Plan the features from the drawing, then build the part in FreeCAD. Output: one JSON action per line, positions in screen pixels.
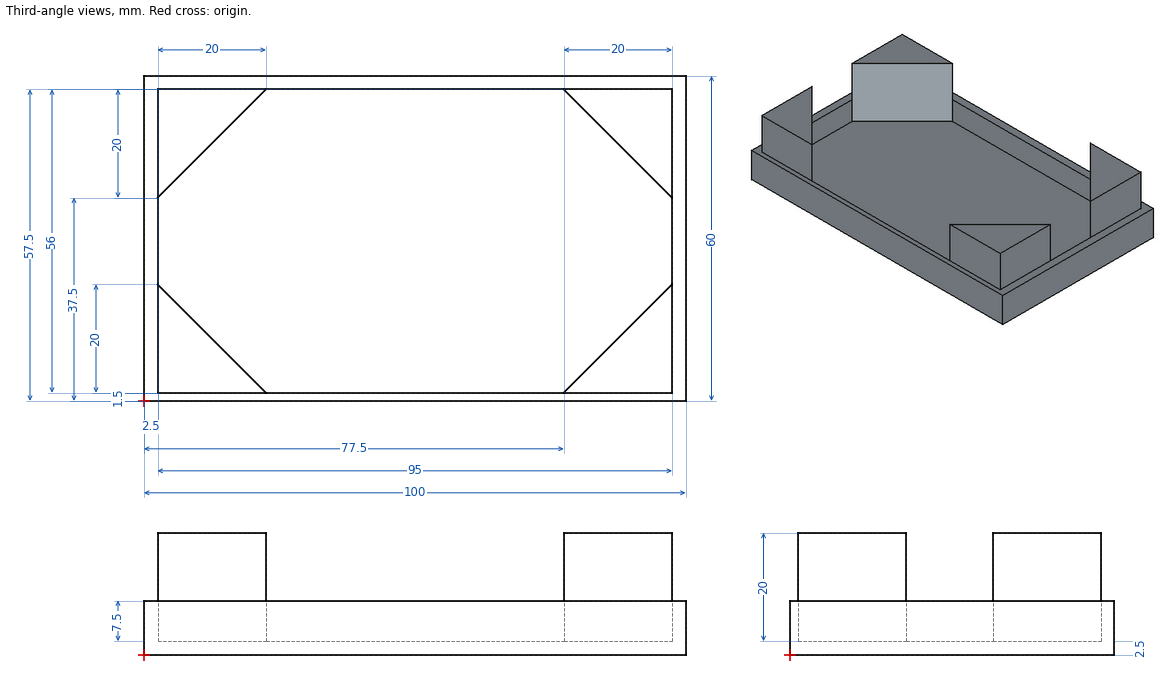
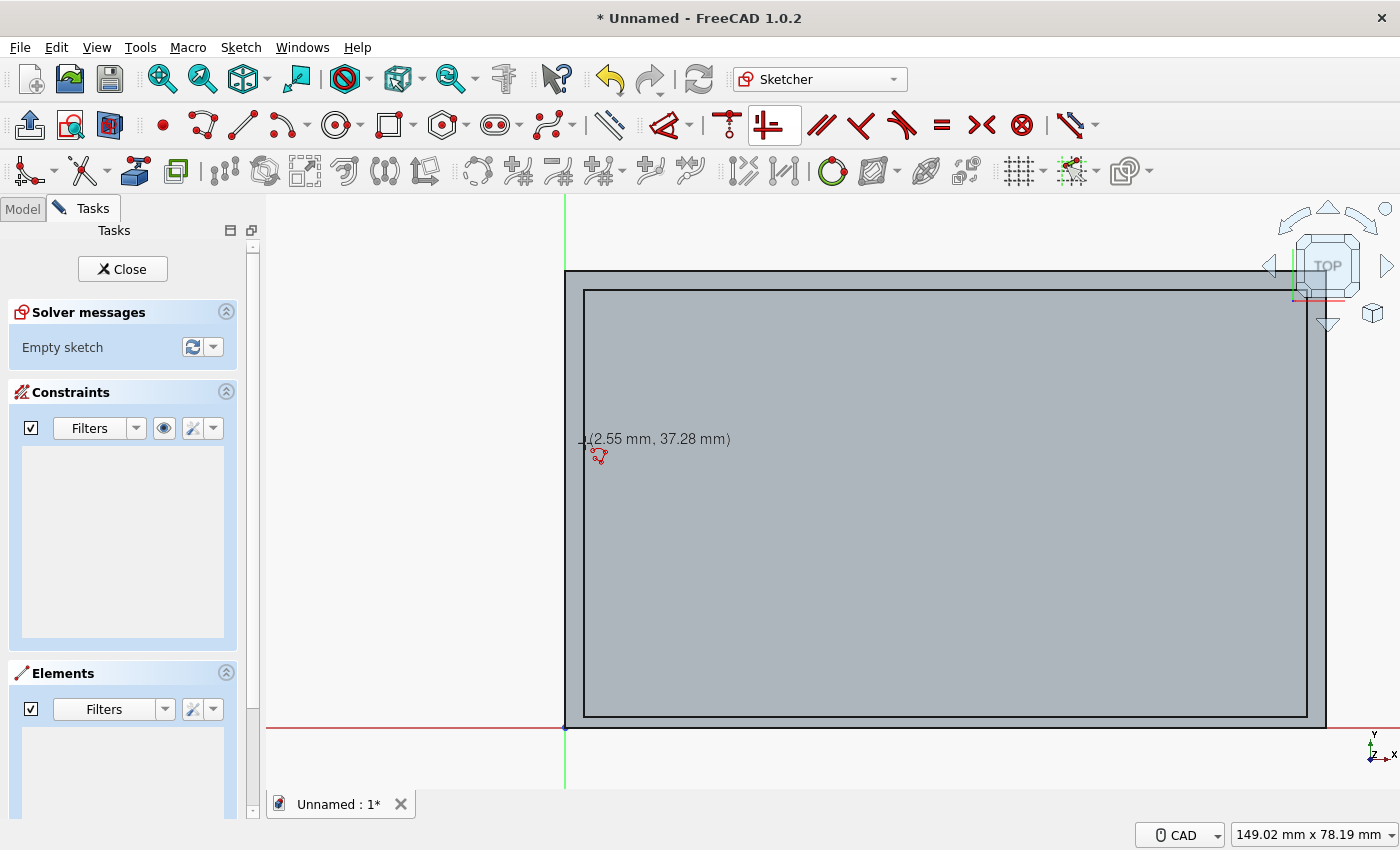
{"action": "left_click", "coordinate": [584, 443]}
{"action": "left_click", "coordinate": [737, 290]}
{"action": "left_click", "coordinate": [584, 290]}
{"action": "left_click", "coordinate": [584, 444]}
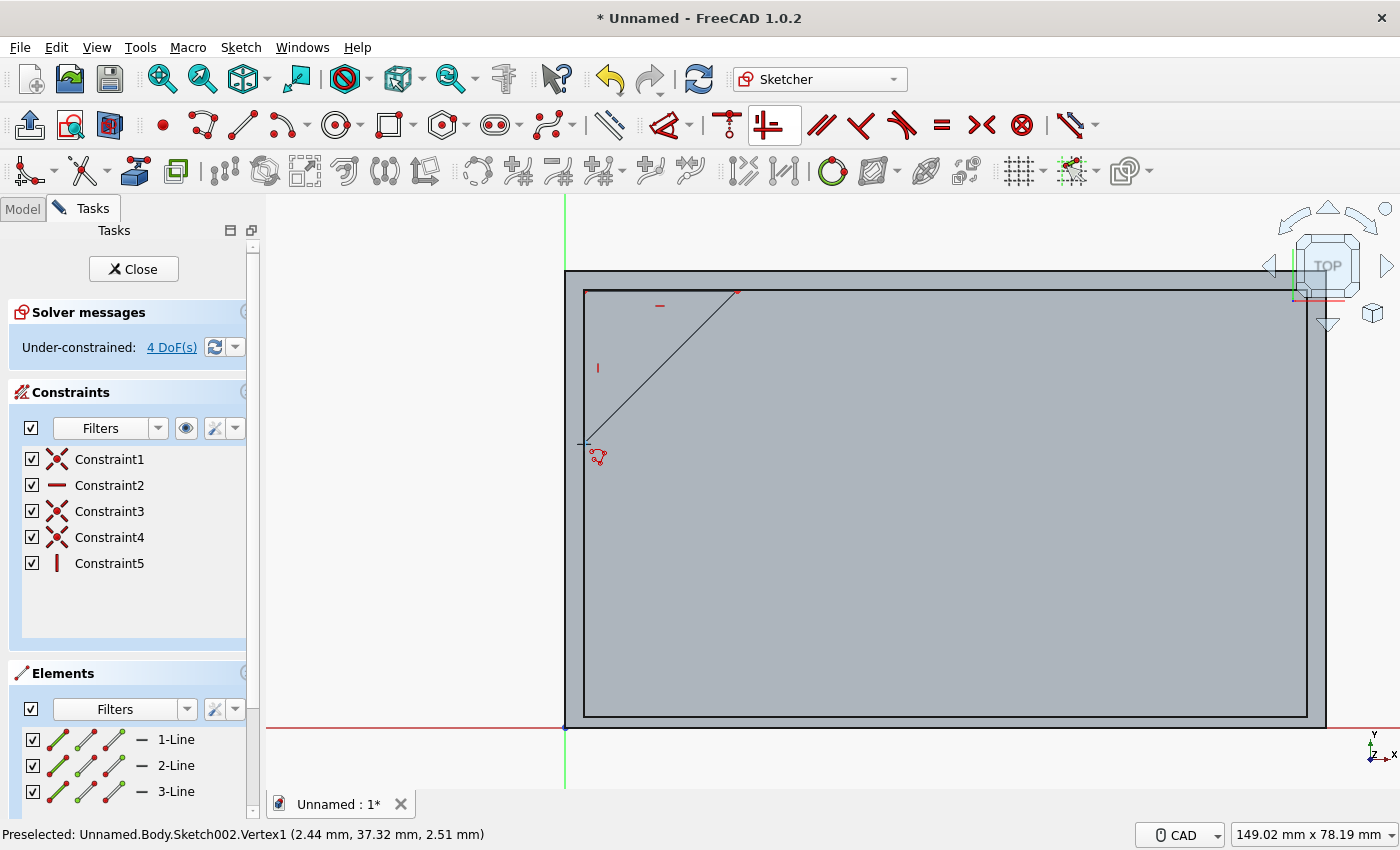
{"action": "scroll", "coordinate": [584, 717], "scroll_direction": "up", "scroll_amount": 2}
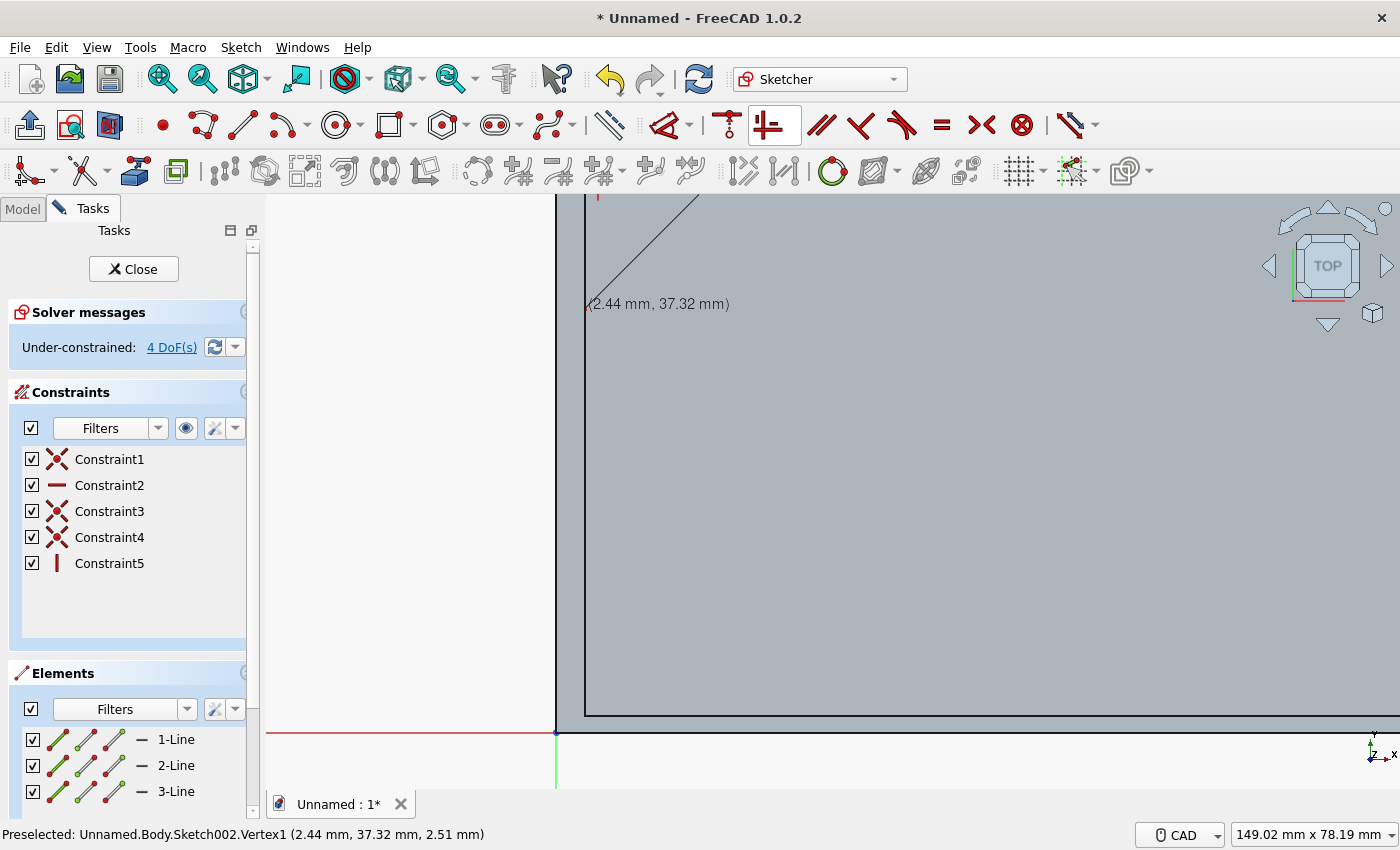
{"action": "left_click", "coordinate": [585, 716]}
{"action": "left_click", "coordinate": [812, 716]}
{"action": "left_click", "coordinate": [585, 489]}
{"action": "left_click", "coordinate": [585, 717]}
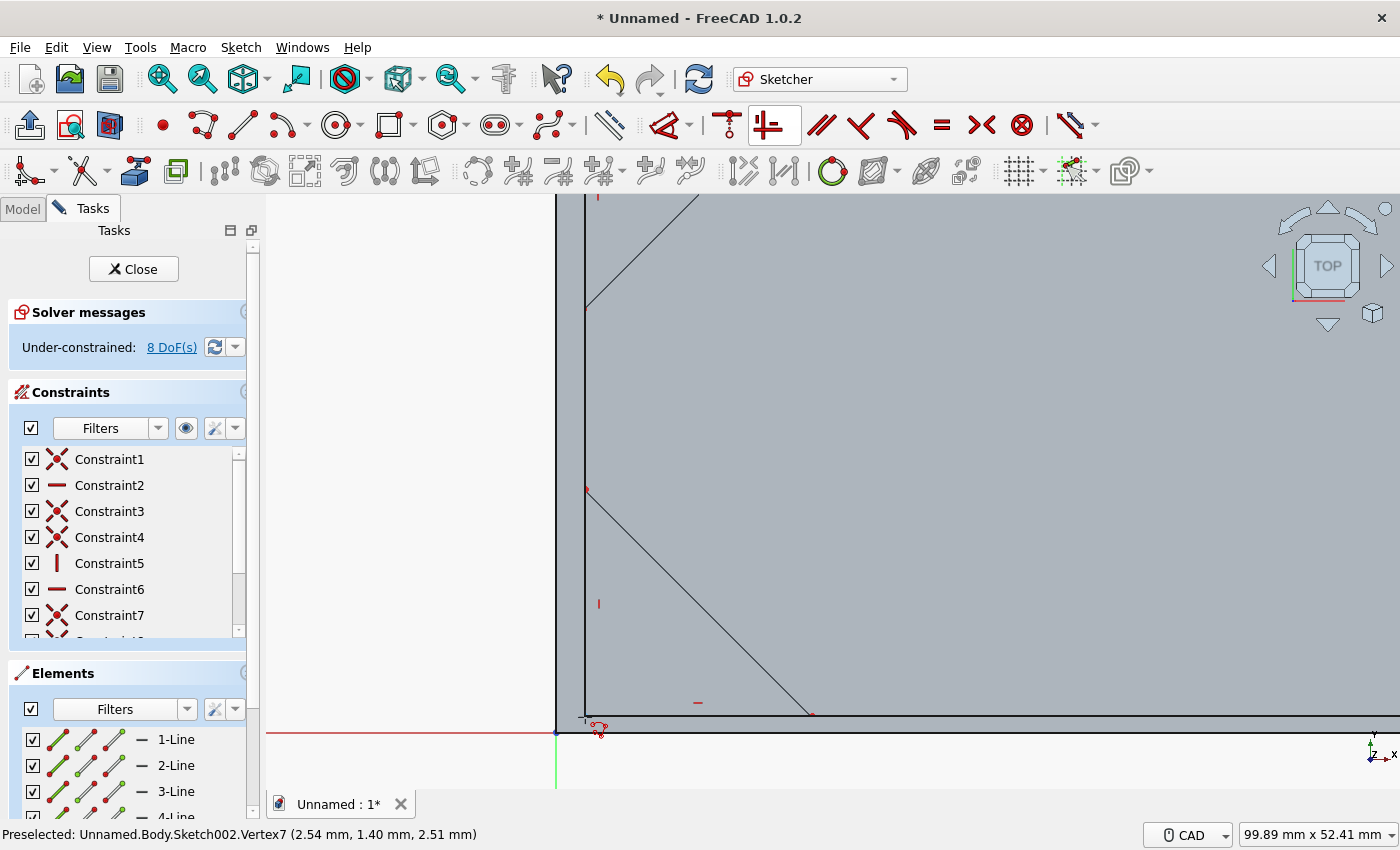
{"action": "scroll", "coordinate": [345, 595], "scroll_direction": "down", "scroll_amount": 3}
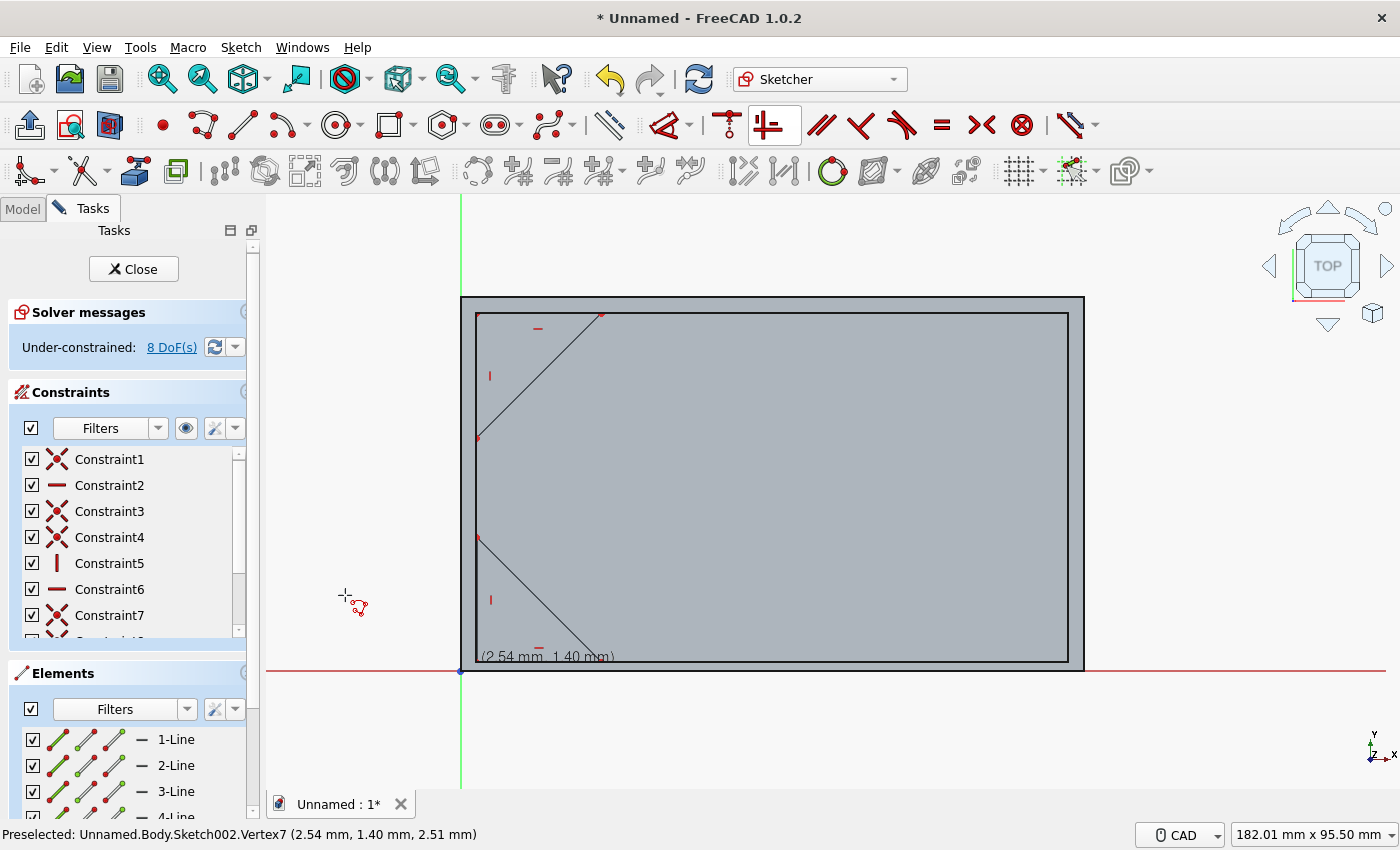
{"action": "left_click", "coordinate": [944, 313]}
{"action": "left_click", "coordinate": [1068, 437]}
{"action": "left_click", "coordinate": [1068, 313]}
{"action": "left_click", "coordinate": [944, 314]}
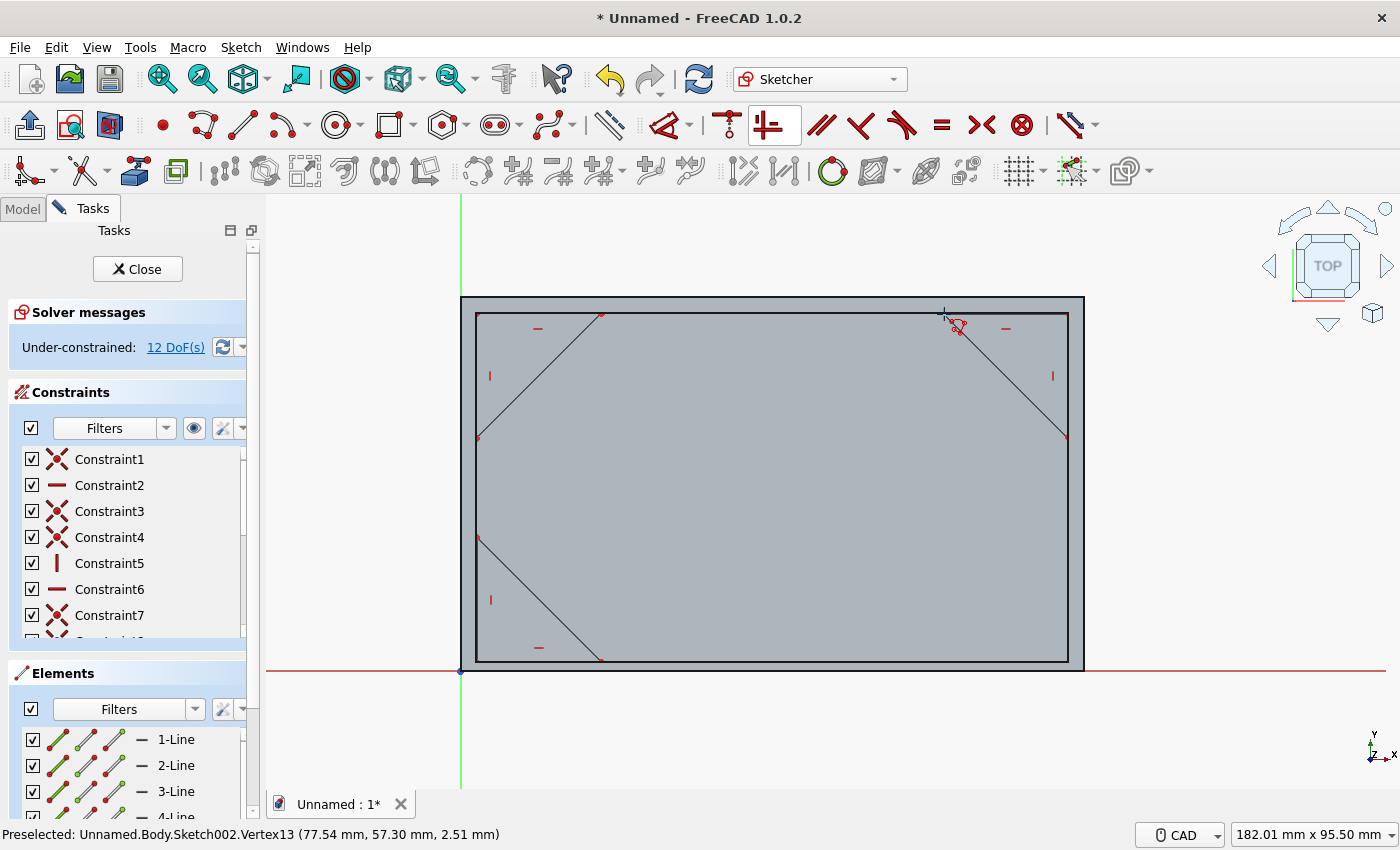
{"action": "scroll", "coordinate": [944, 662], "scroll_direction": "up", "scroll_amount": 3}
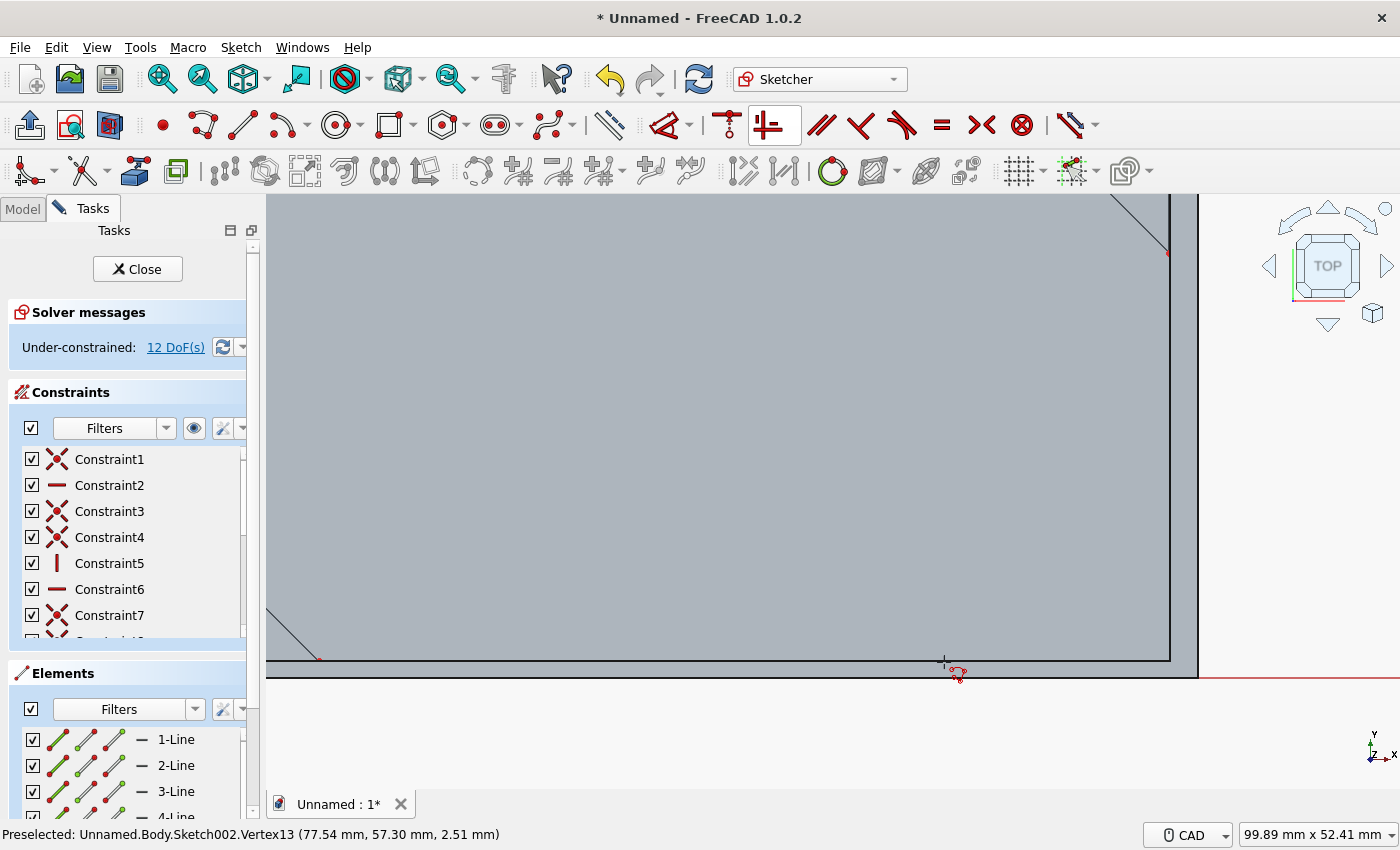
{"action": "left_click", "coordinate": [943, 661]}
{"action": "left_click", "coordinate": [1170, 661]}
{"action": "left_click", "coordinate": [1170, 434]}
{"action": "left_click", "coordinate": [943, 662]}
{"action": "key", "text": "Escape"}
{"action": "key", "text": "Escape"}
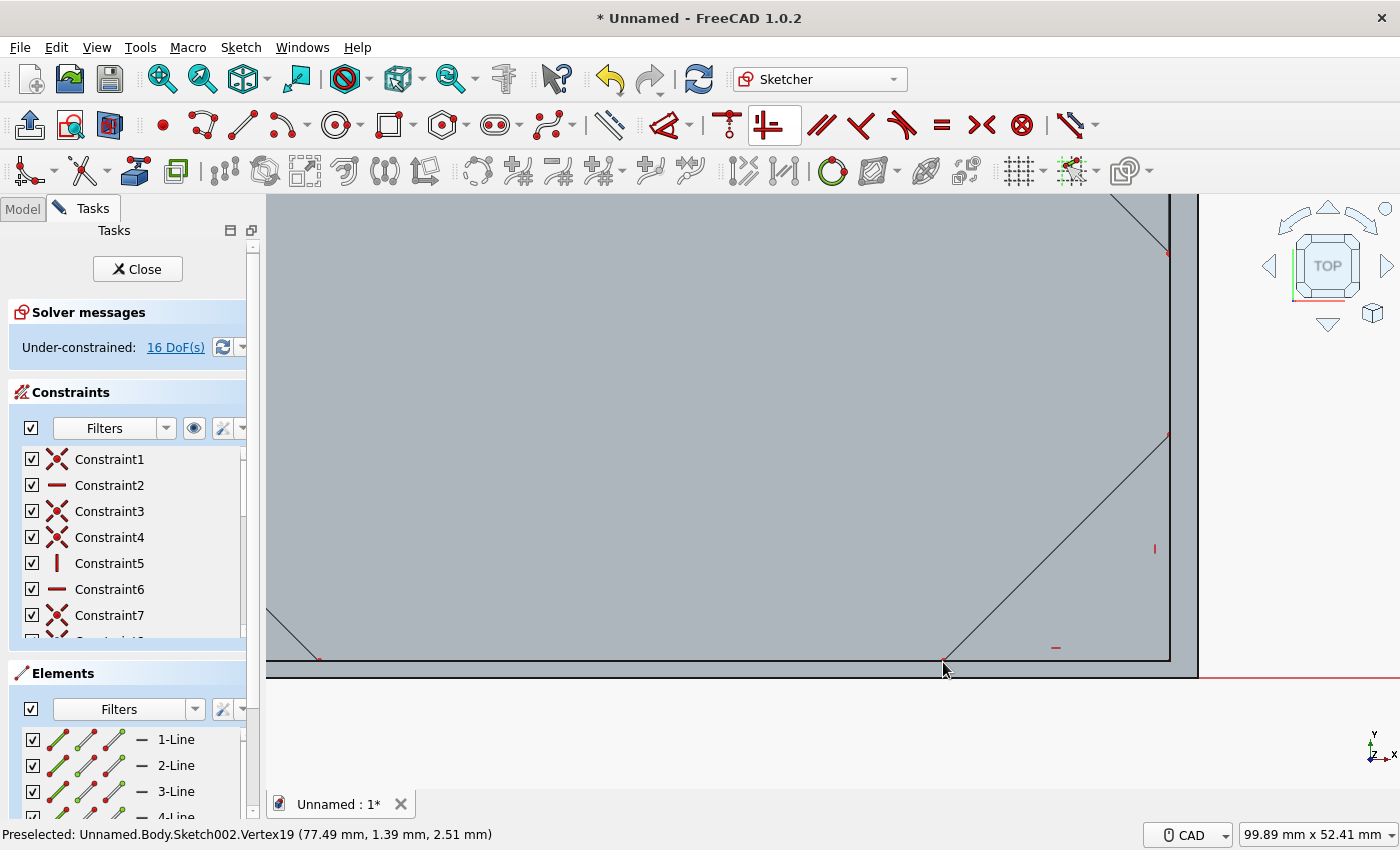
{"action": "left_click", "coordinate": [664, 126]}